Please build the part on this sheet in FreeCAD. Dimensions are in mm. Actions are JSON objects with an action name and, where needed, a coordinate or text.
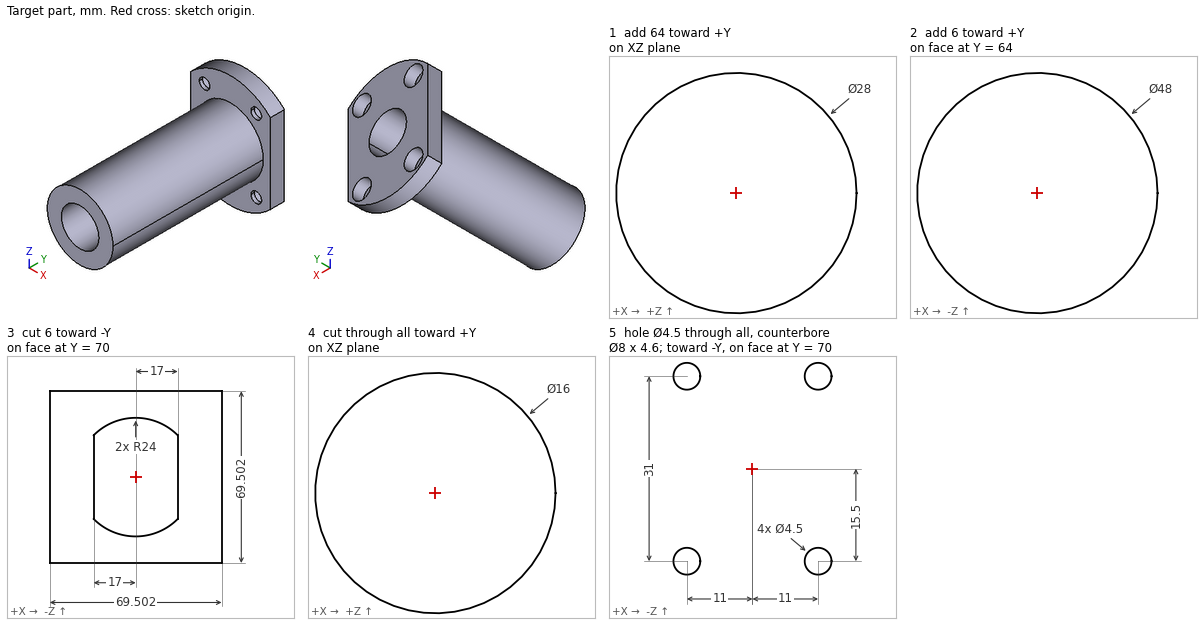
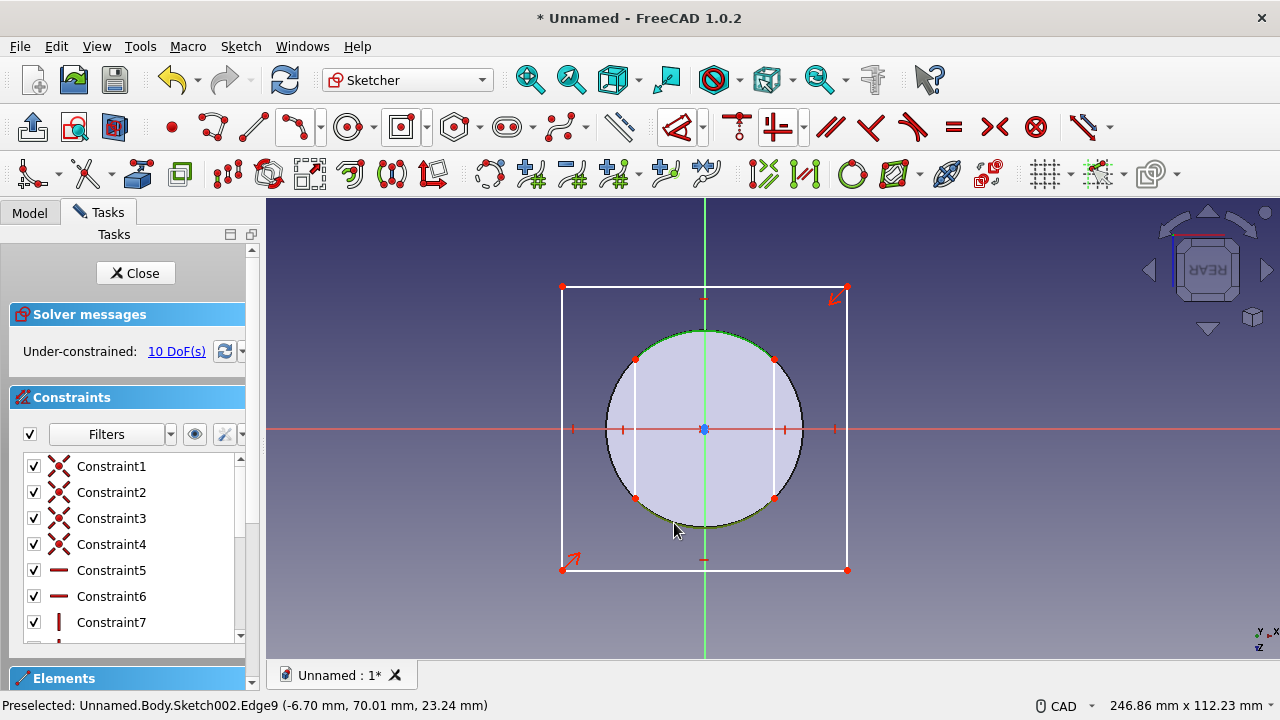
{"action": "left_click", "coordinate": [737, 128]}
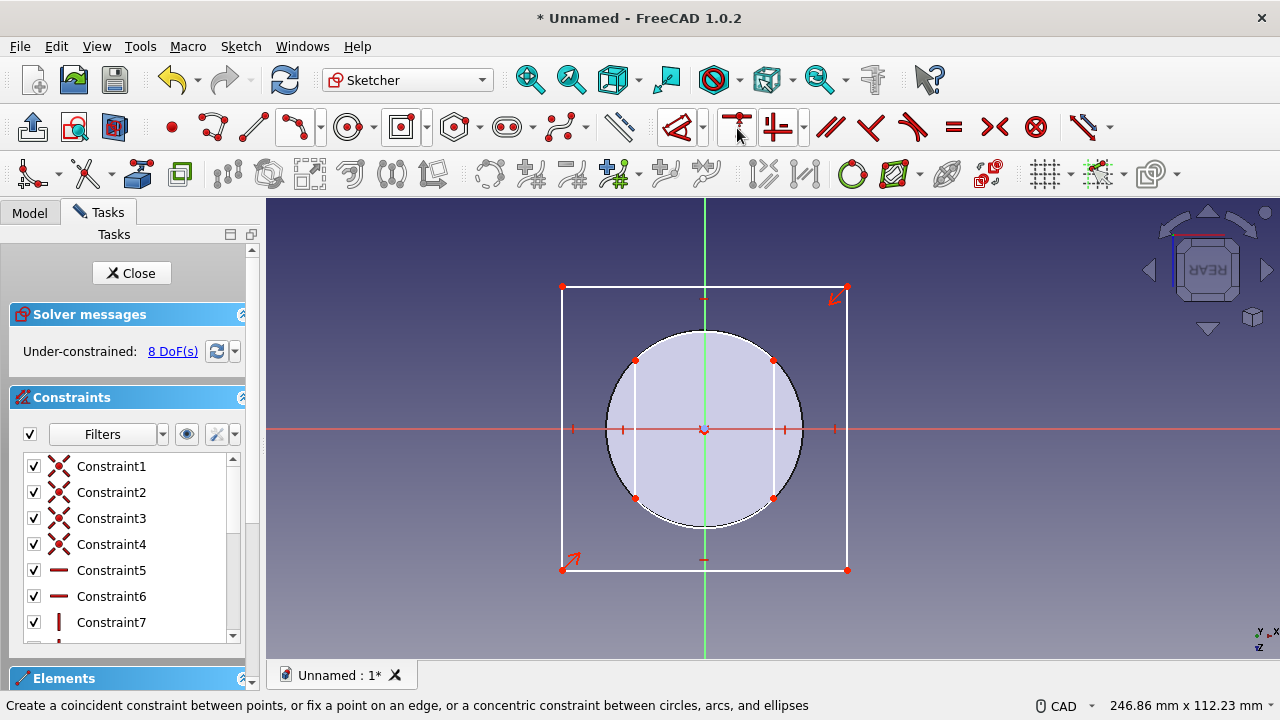
{"action": "left_click_drag", "start_coordinate": [695, 419], "coordinate": [715, 441]}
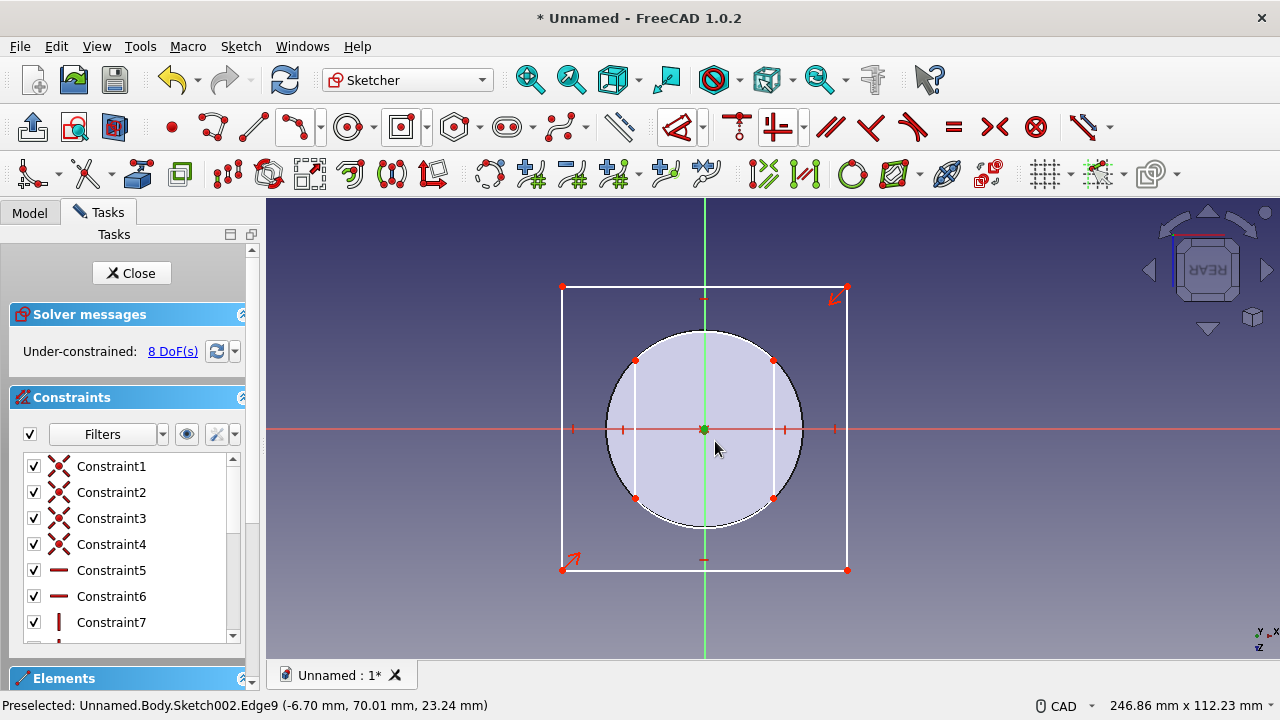
{"action": "key", "text": "c"}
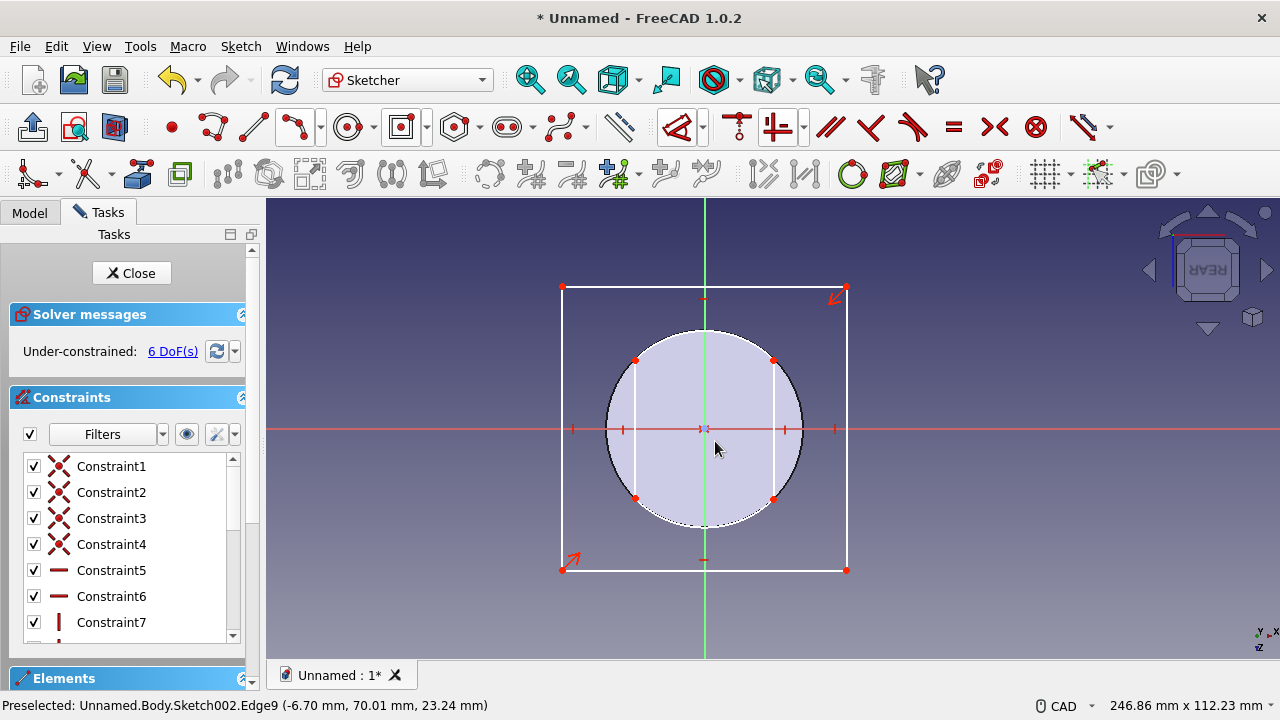
{"action": "left_click", "coordinate": [735, 336]}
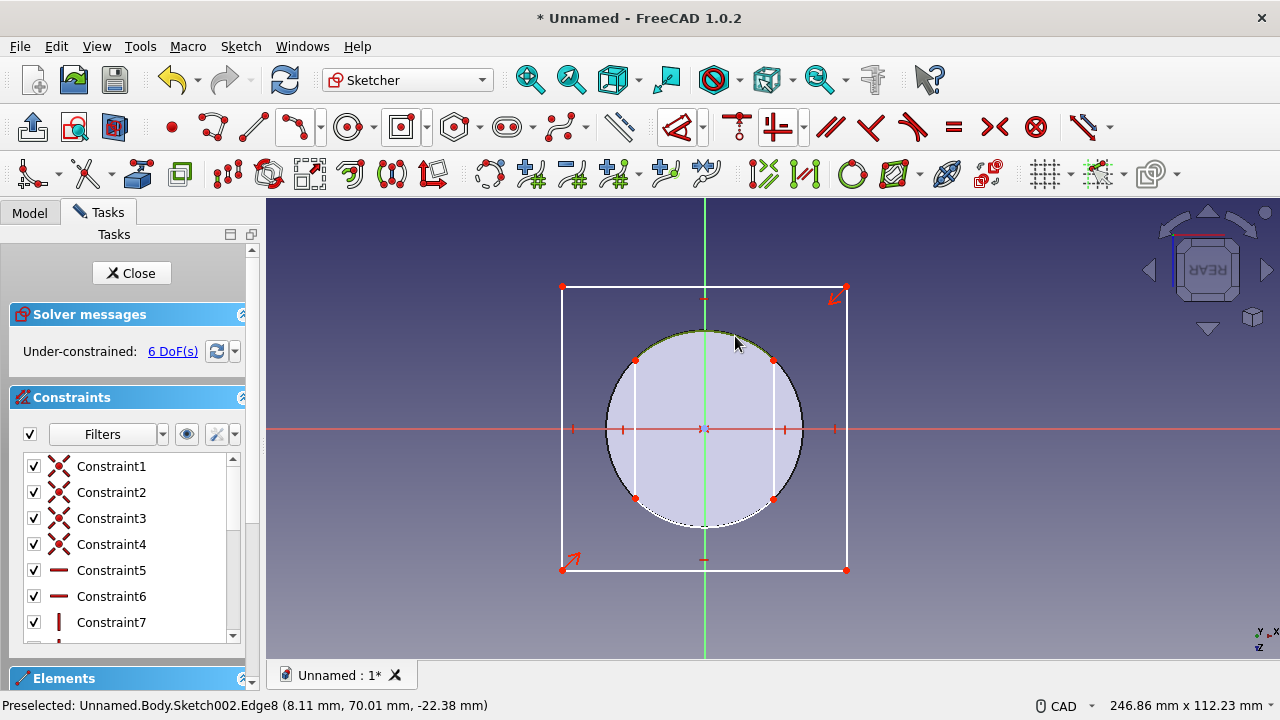
{"action": "left_click", "coordinate": [674, 523]}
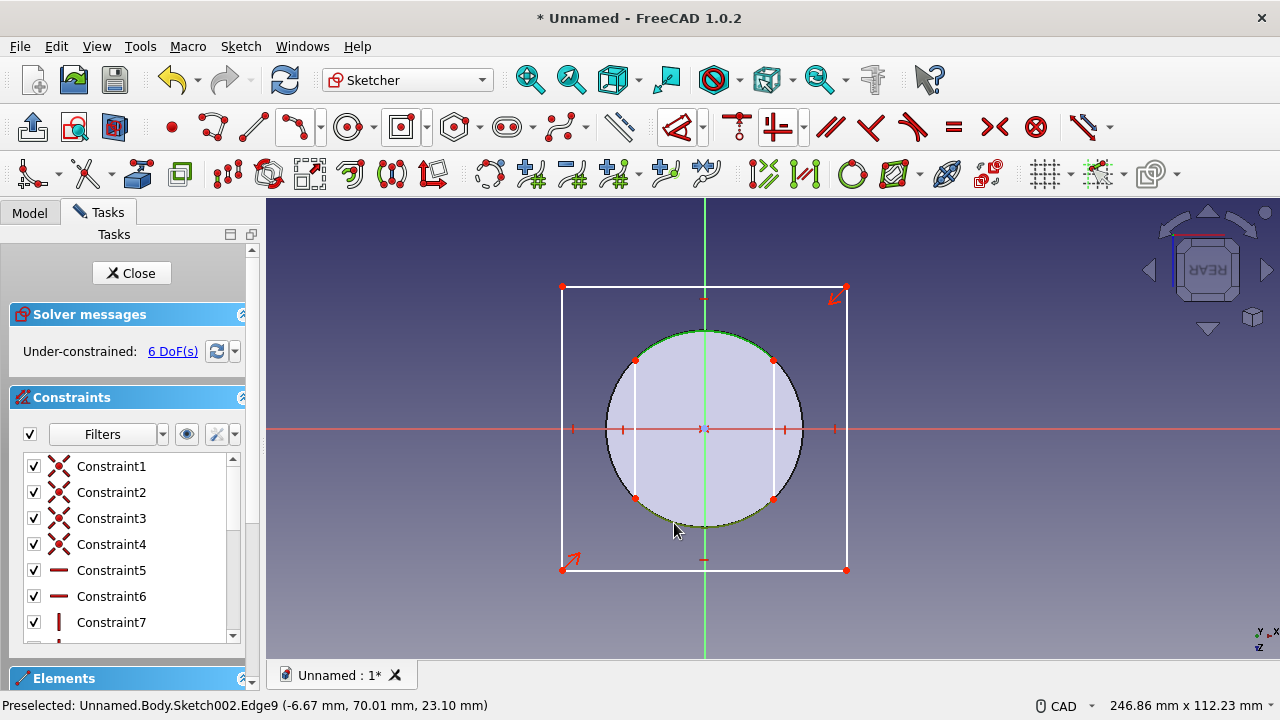
{"action": "left_click", "coordinate": [954, 128]}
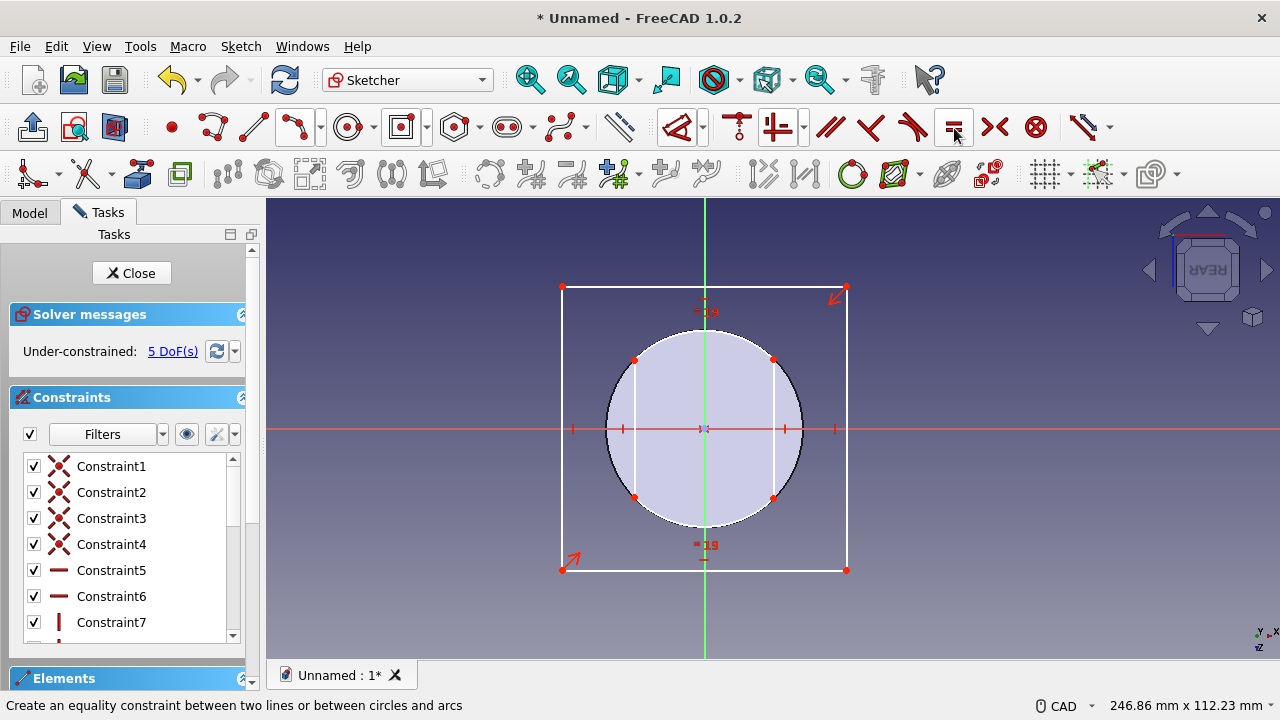
{"action": "left_click", "coordinate": [735, 336]}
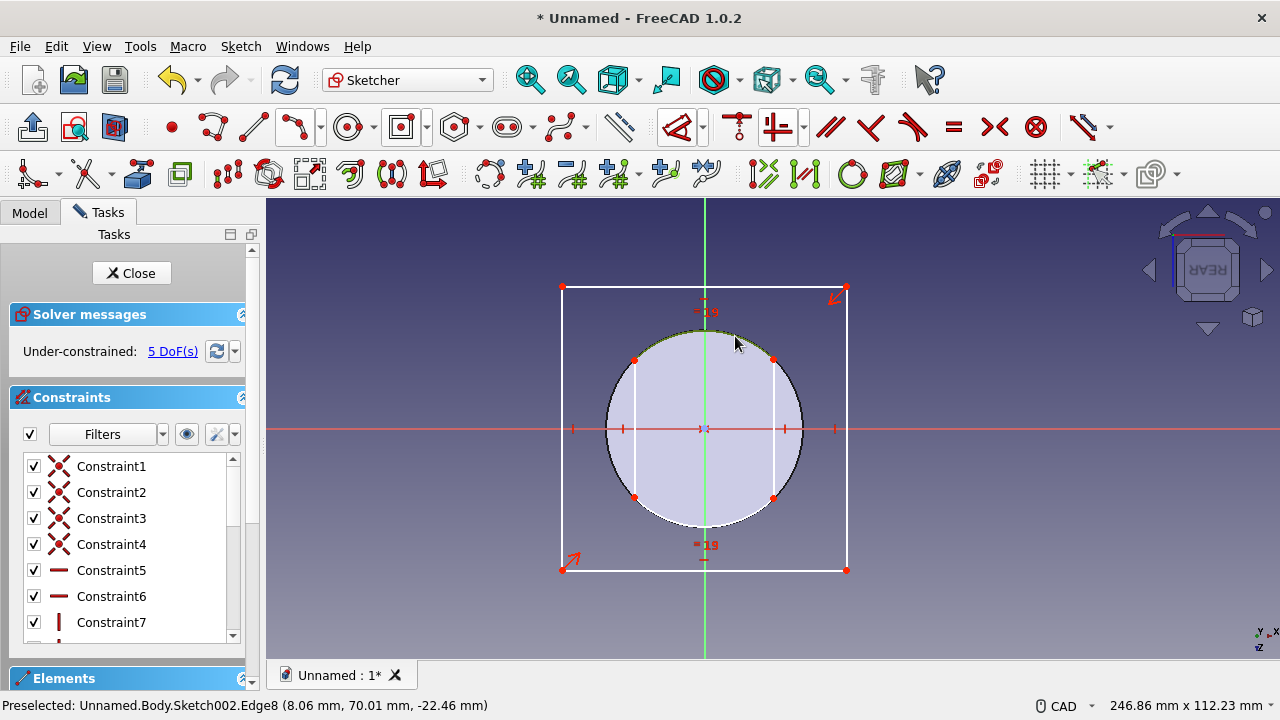
{"action": "left_click", "coordinate": [702, 128]}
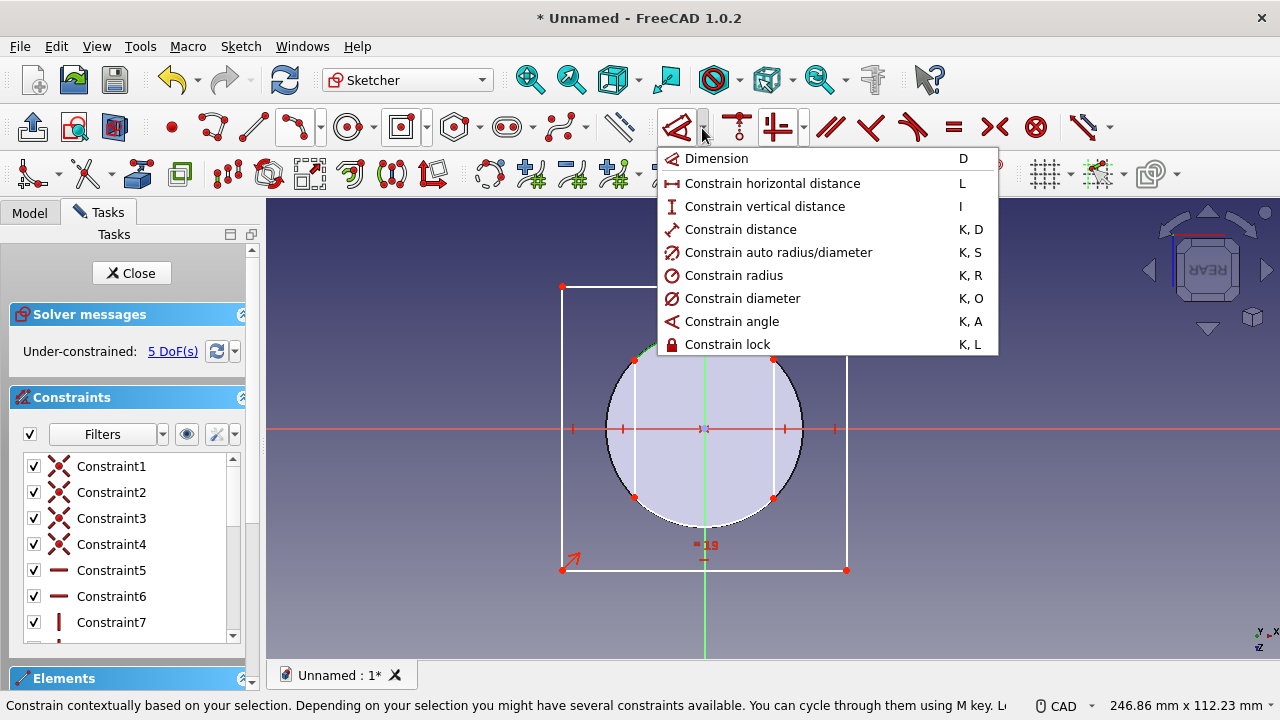
{"action": "left_click", "coordinate": [828, 276]}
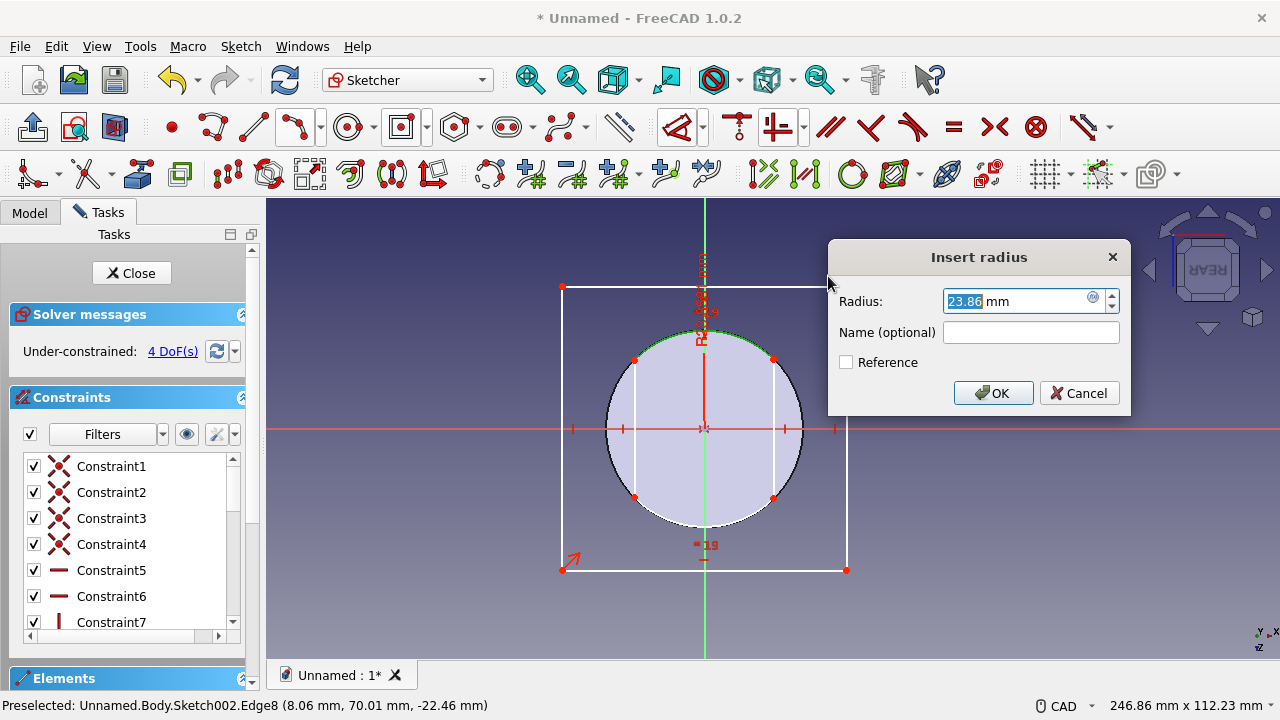
{"action": "type", "text": "24"}
{"action": "key", "text": "Return"}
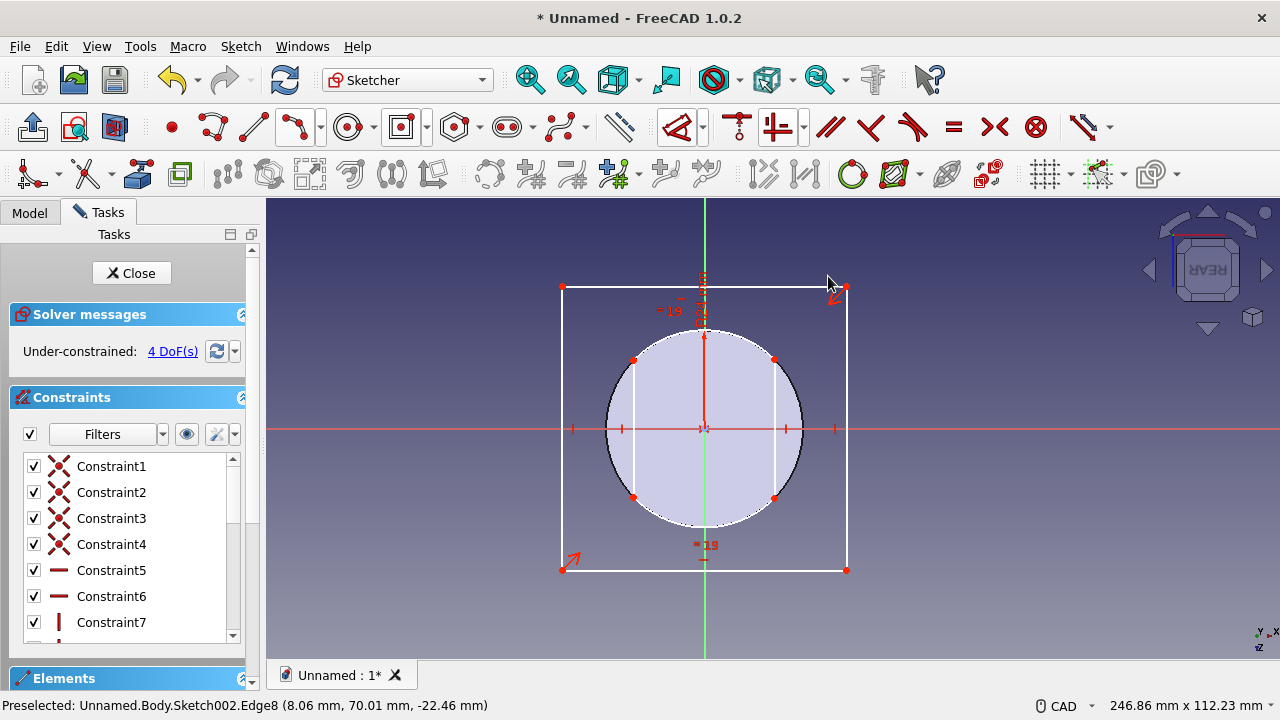
{"action": "left_click", "coordinate": [634, 498]}